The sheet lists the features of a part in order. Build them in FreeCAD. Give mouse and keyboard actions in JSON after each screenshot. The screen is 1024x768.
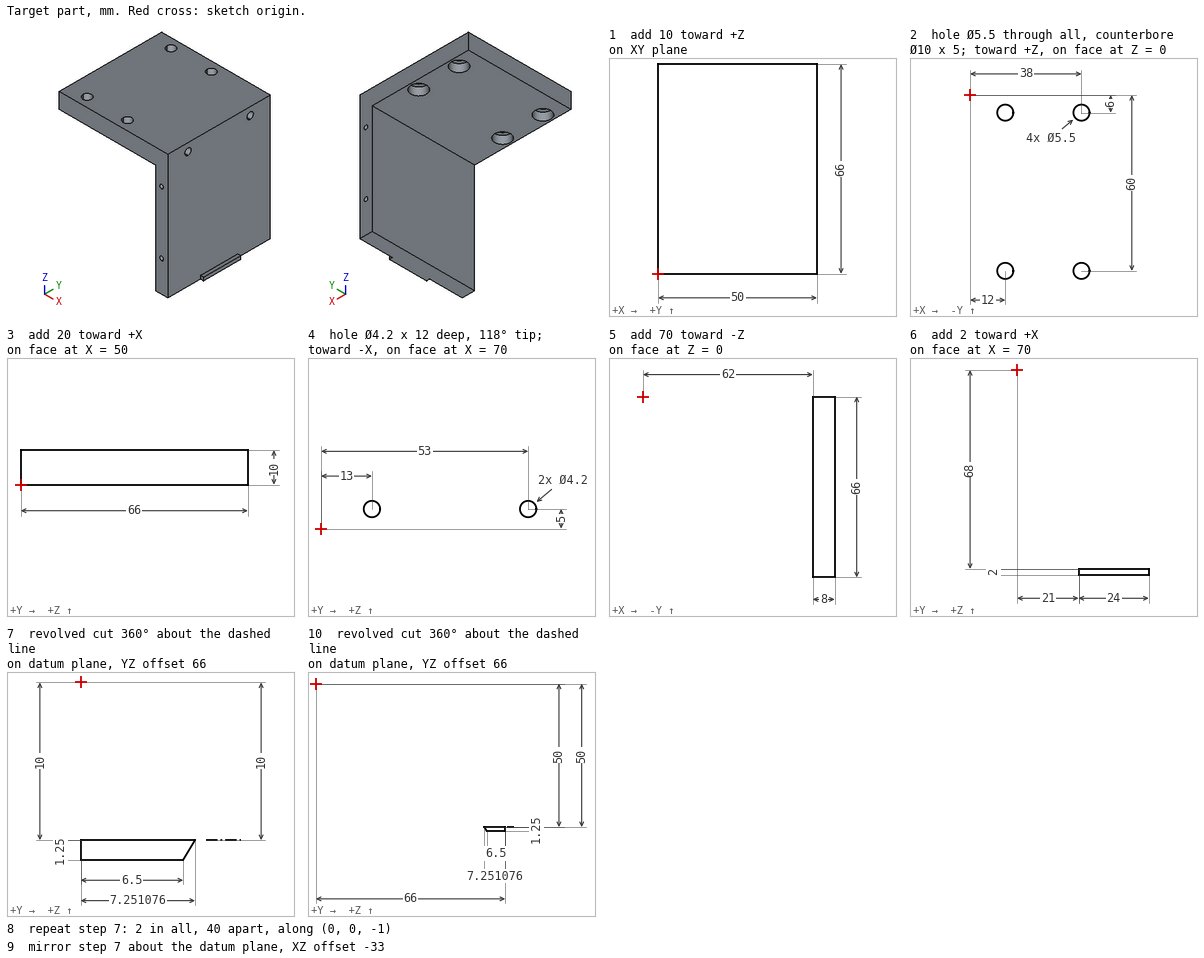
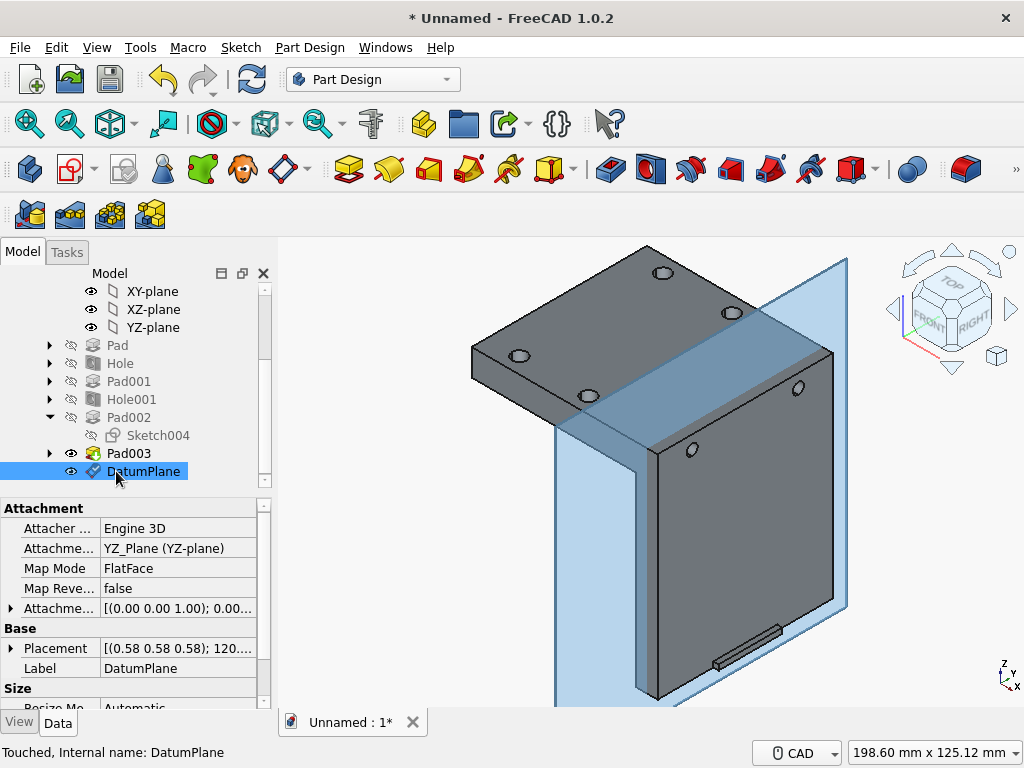
{"action": "left_click", "coordinate": [70, 170]}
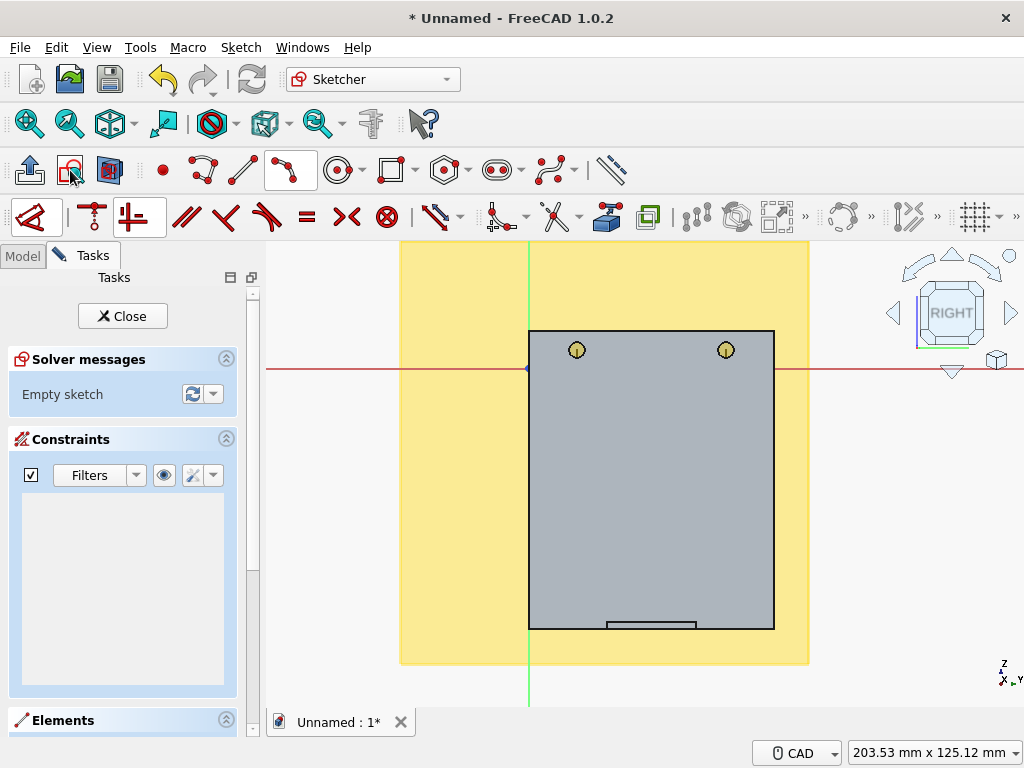
{"action": "key", "text": "q s"}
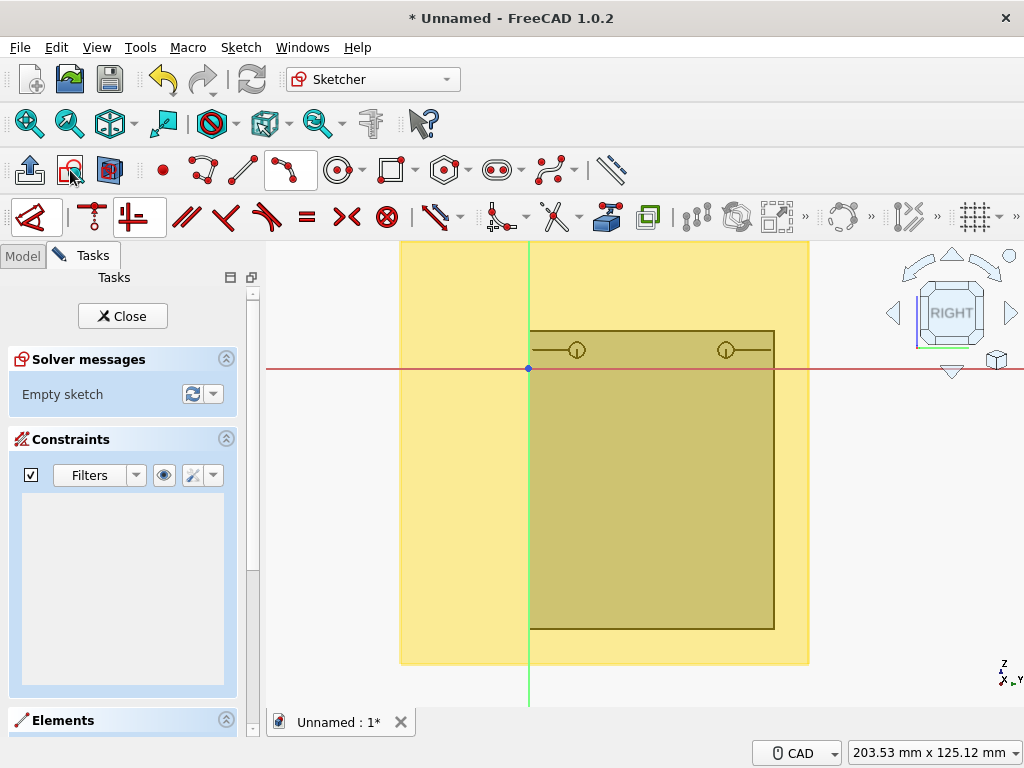
{"action": "scroll", "coordinate": [543, 376], "scroll_direction": "up", "scroll_amount": 10}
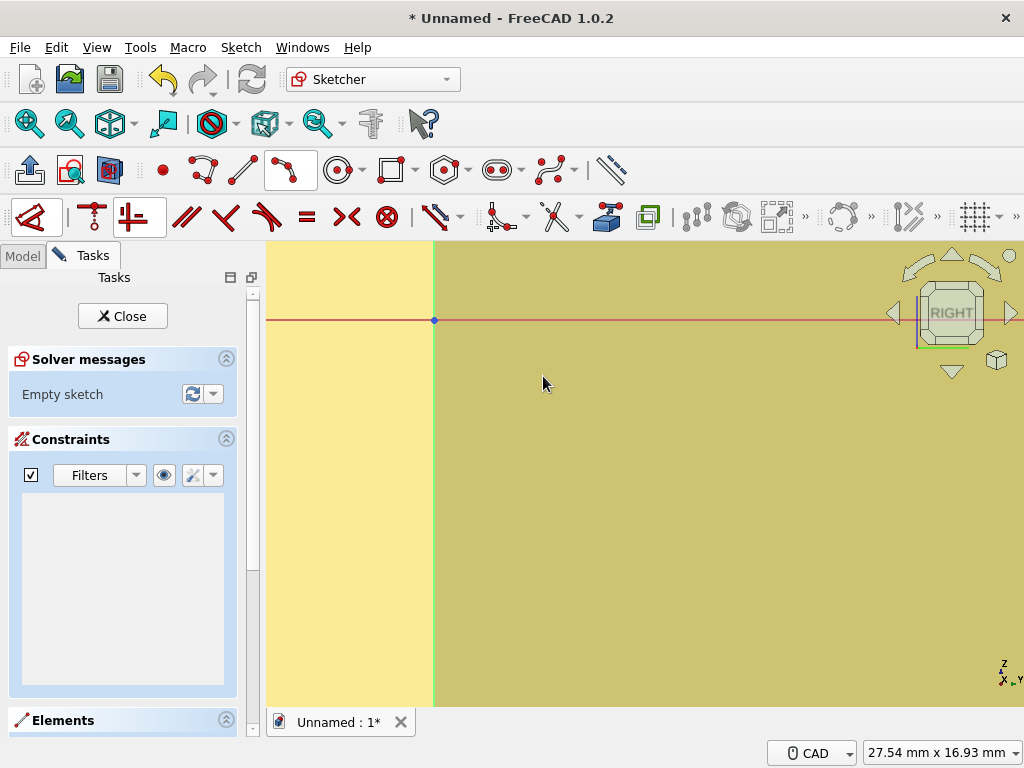
{"action": "key", "text": "g m"}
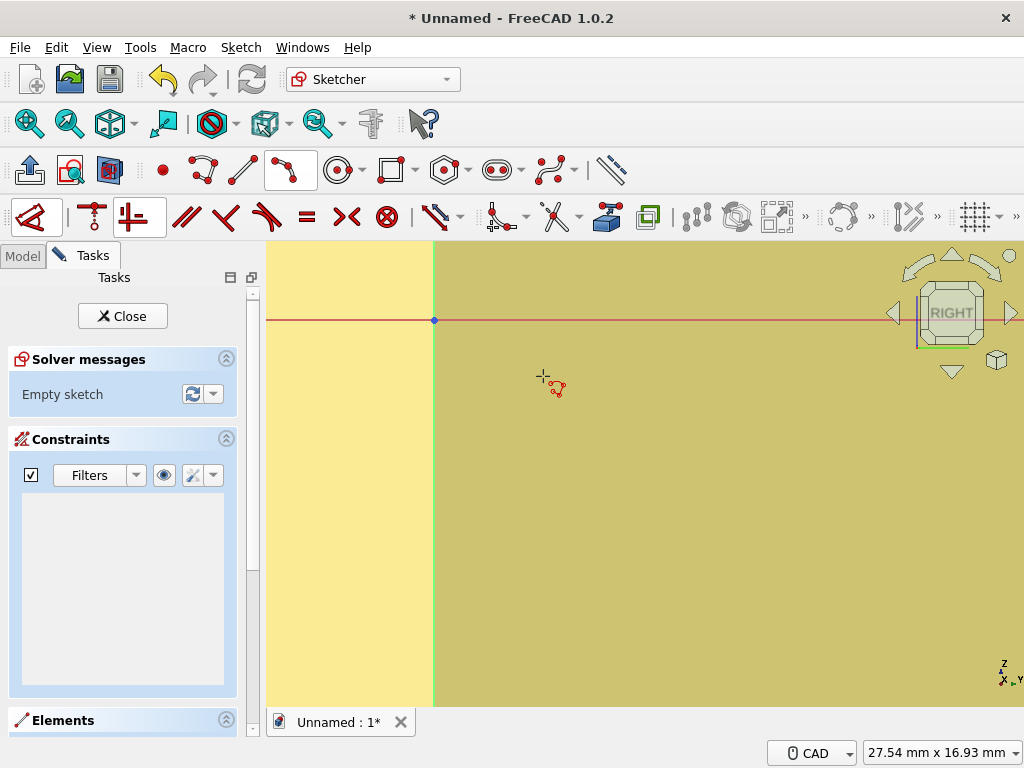
{"action": "left_click", "coordinate": [434, 596]}
{"action": "left_click", "coordinate": [443, 630]}
{"action": "left_click", "coordinate": [613, 630]}
{"action": "left_click", "coordinate": [634, 596]}
{"action": "left_click", "coordinate": [434, 597]}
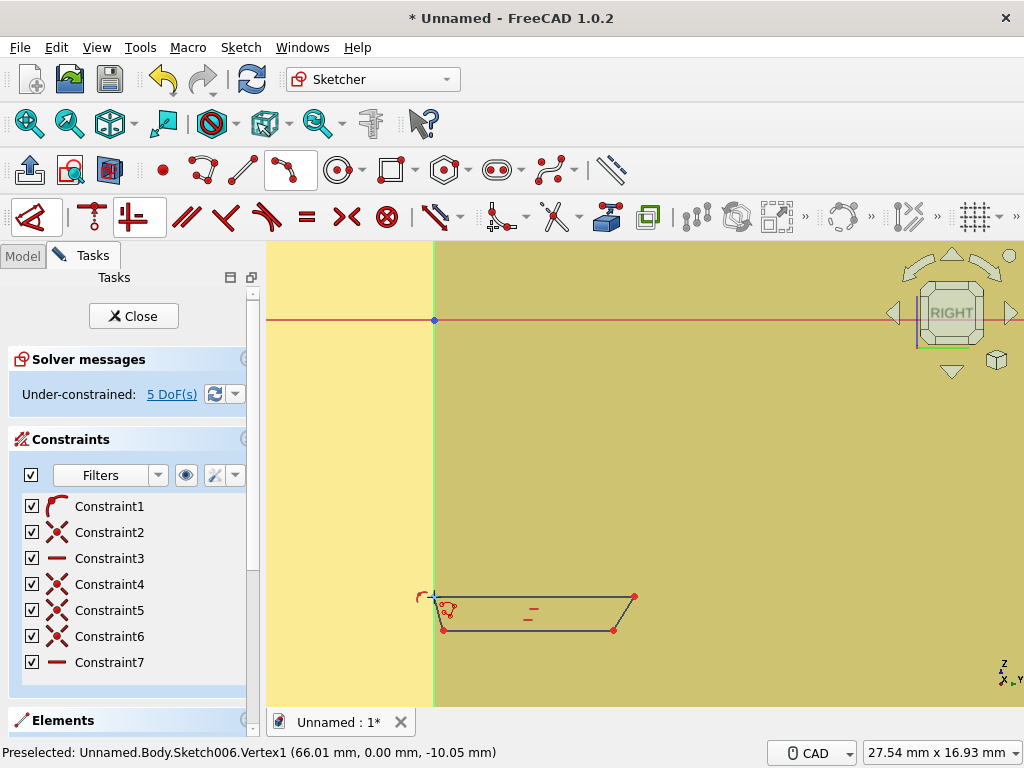
{"action": "key", "text": "g l"}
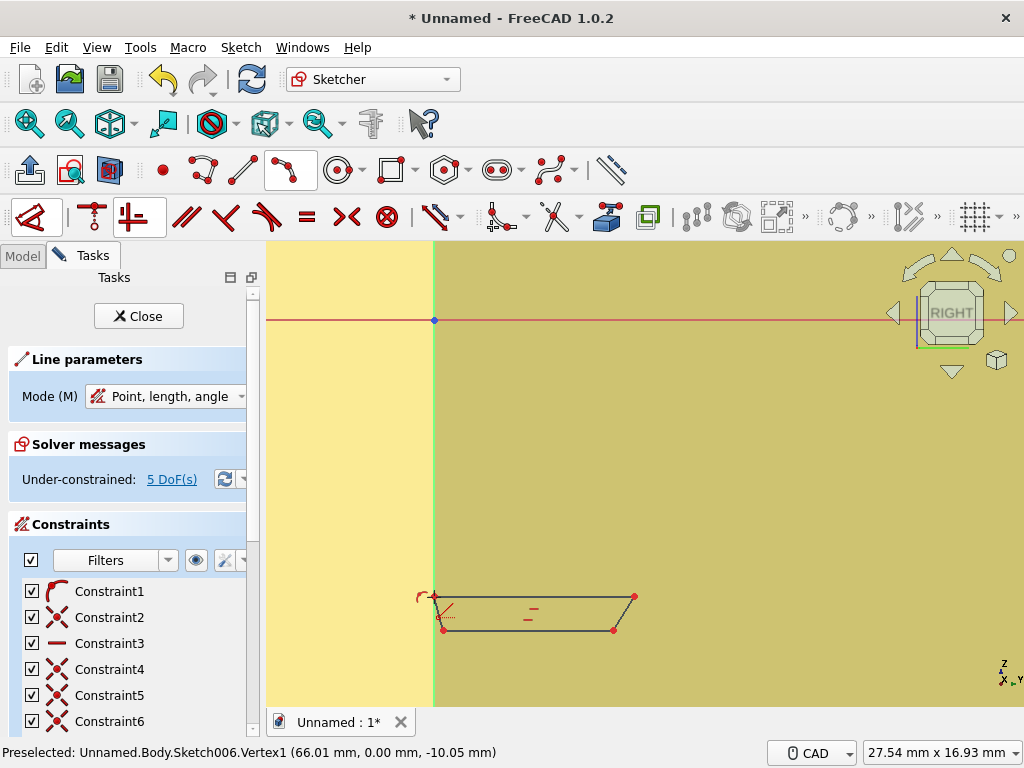
{"action": "left_click", "coordinate": [654, 596]}
{"action": "left_click", "coordinate": [713, 596]}
{"action": "key", "text": "Escape"}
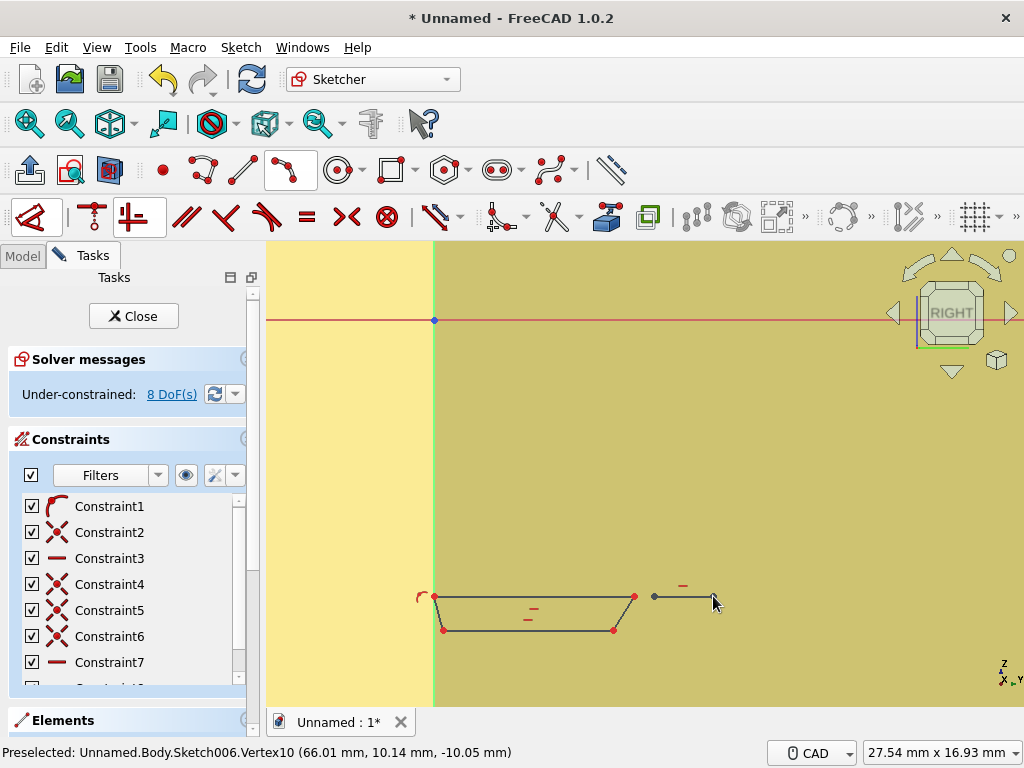
{"action": "left_click", "coordinate": [672, 597]}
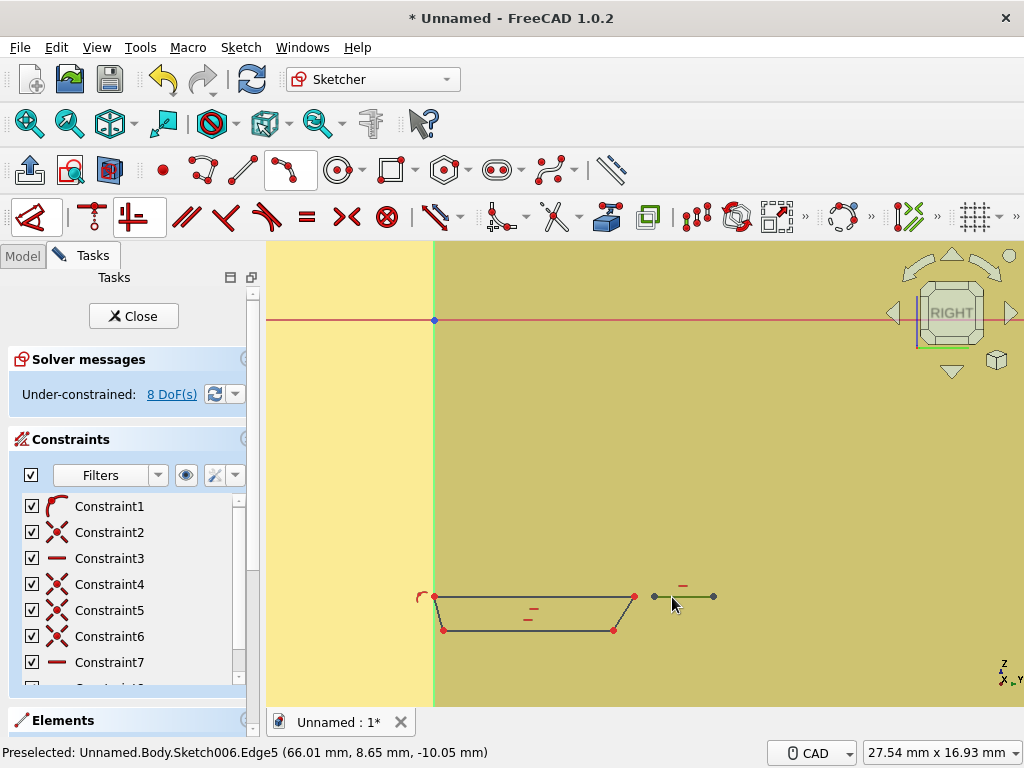
{"action": "left_click", "coordinate": [612, 170]}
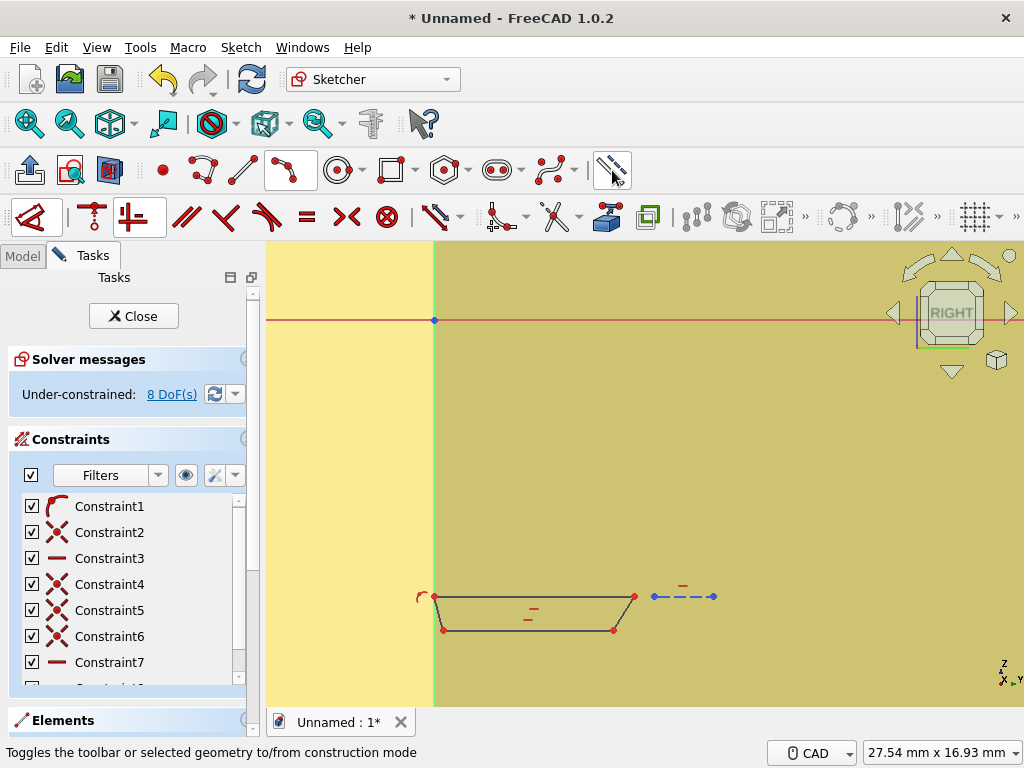
{"action": "scroll", "coordinate": [437, 607], "scroll_direction": "up", "scroll_amount": 2}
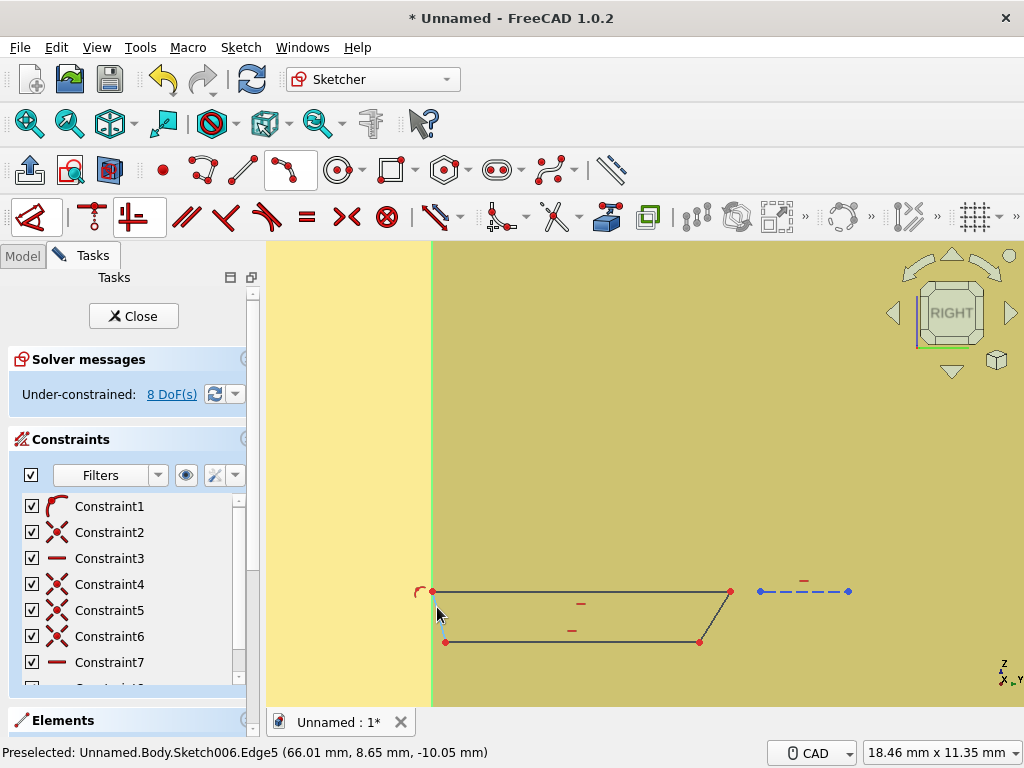
{"action": "left_click", "coordinate": [436, 607]}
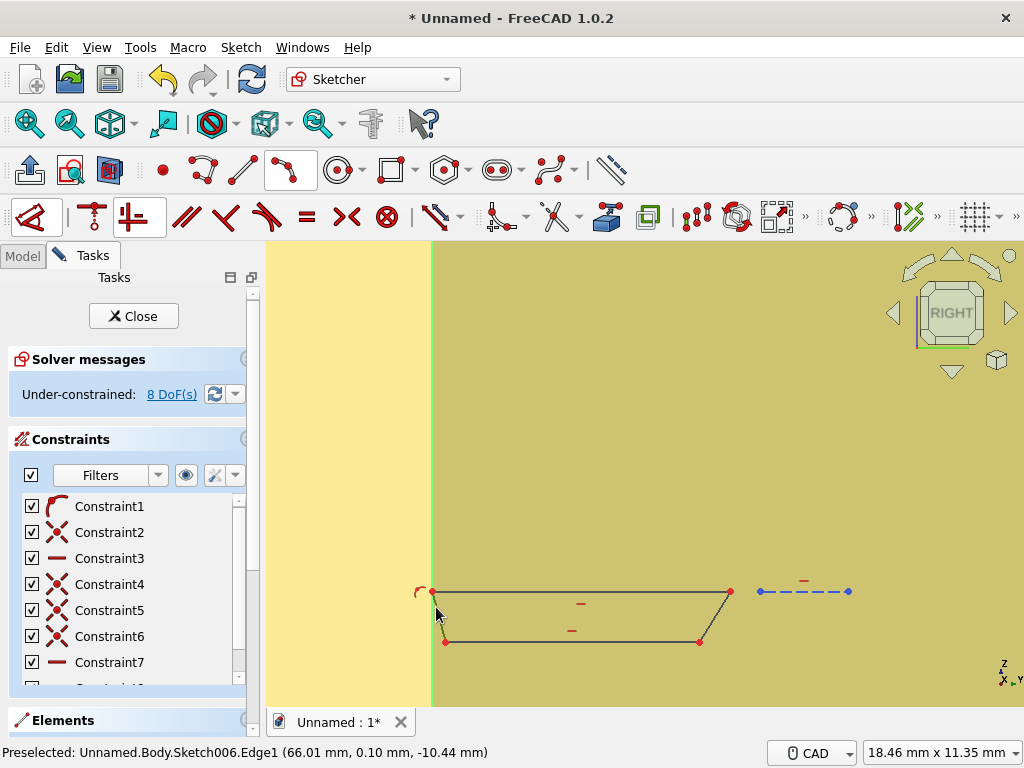
{"action": "key", "text": "v"}